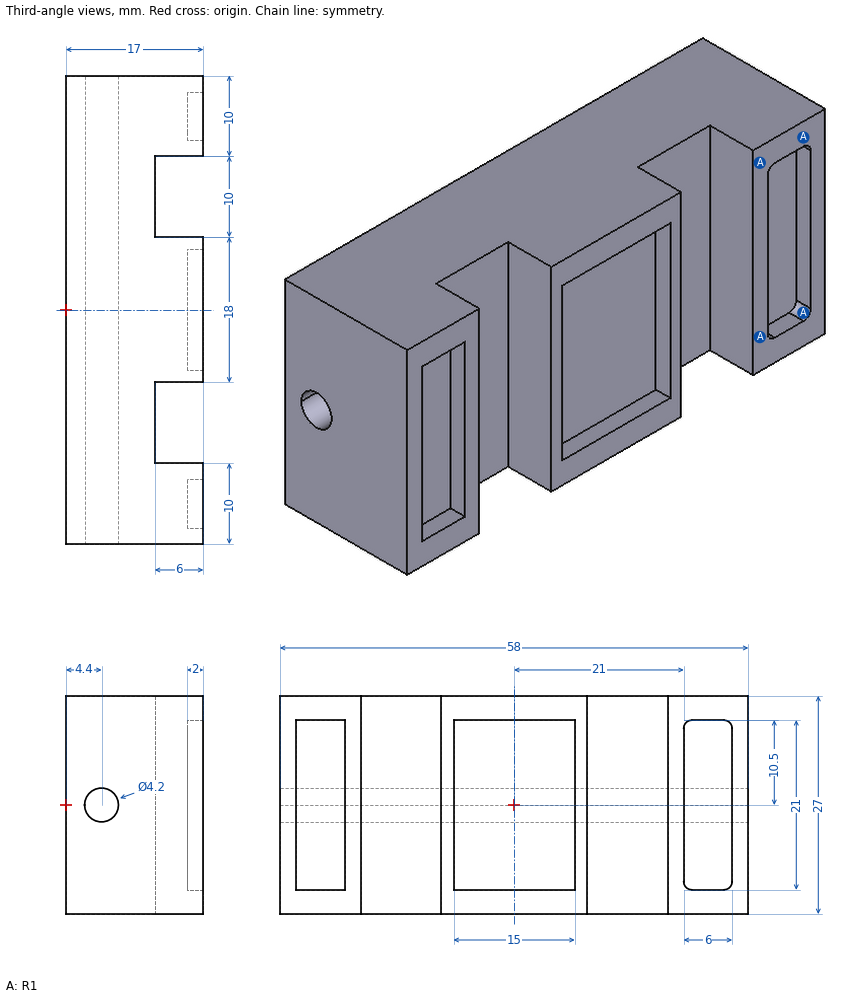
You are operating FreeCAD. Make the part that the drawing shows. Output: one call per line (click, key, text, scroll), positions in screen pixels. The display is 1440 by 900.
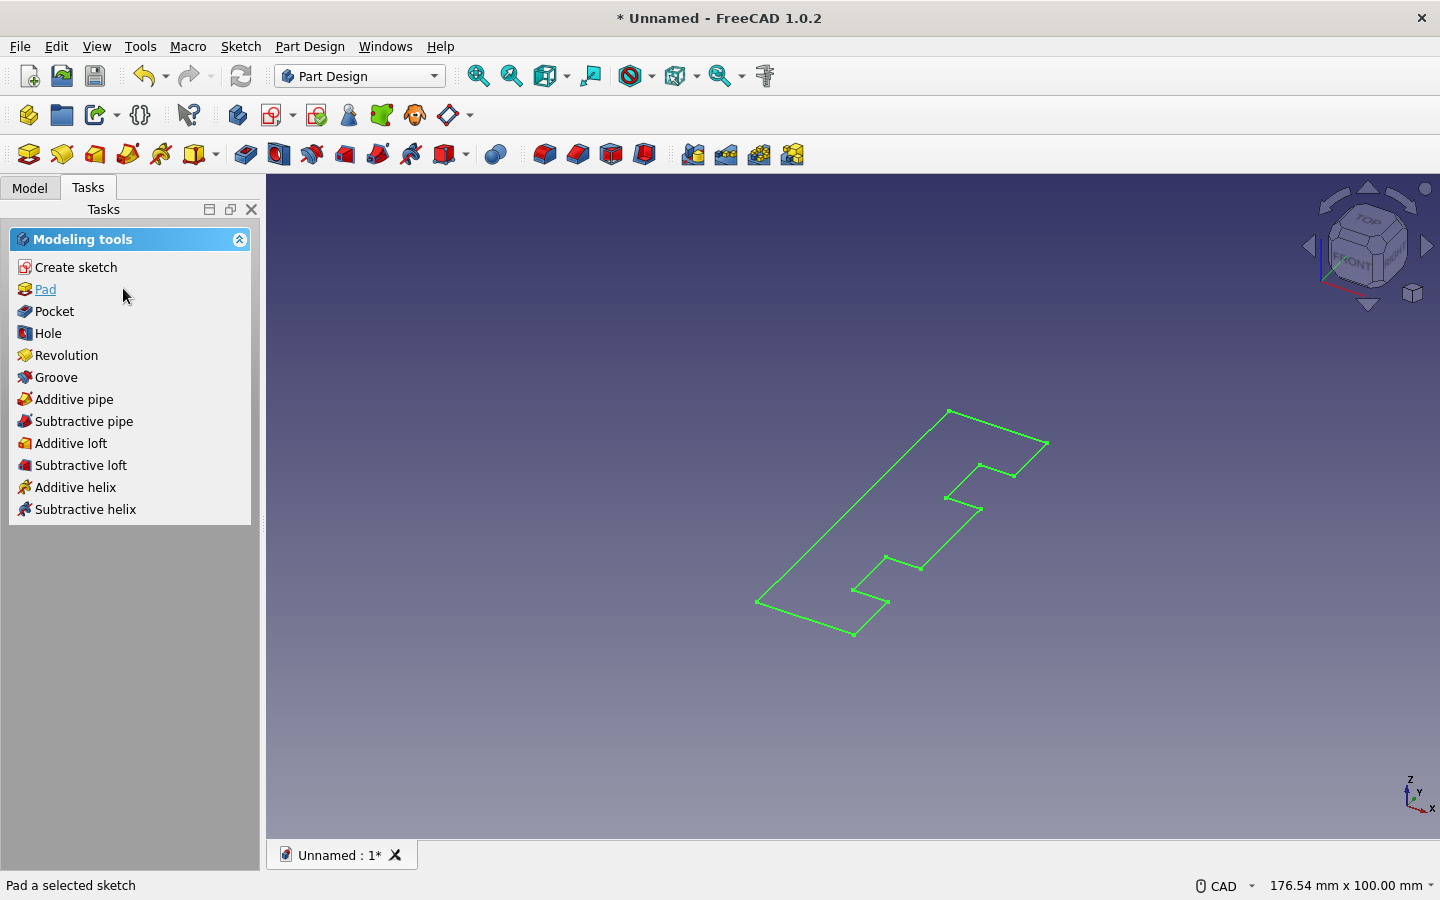
click(29, 154)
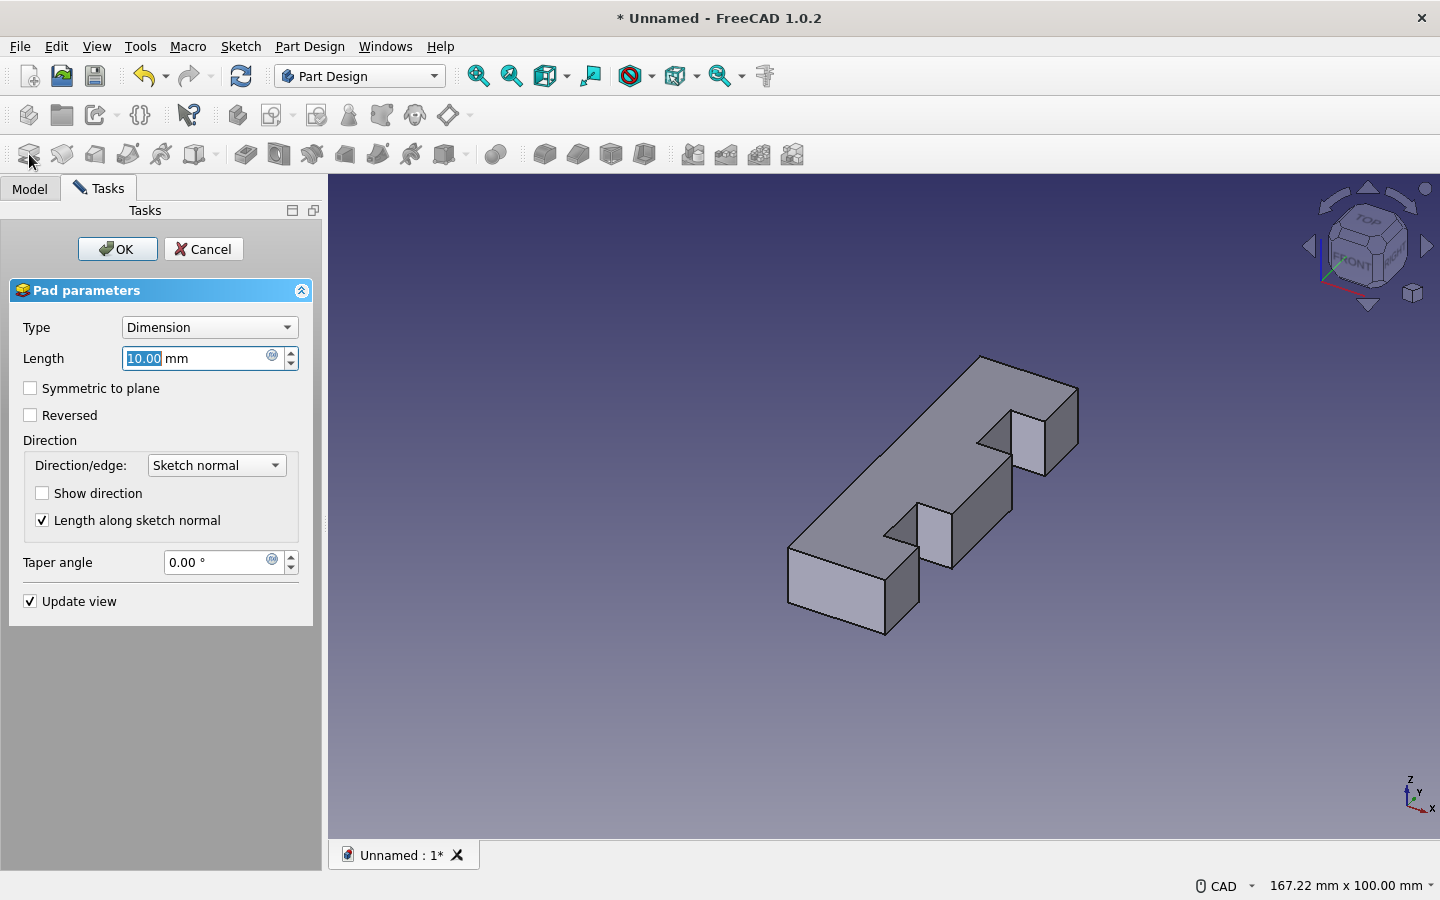
text(27)
key(Tab)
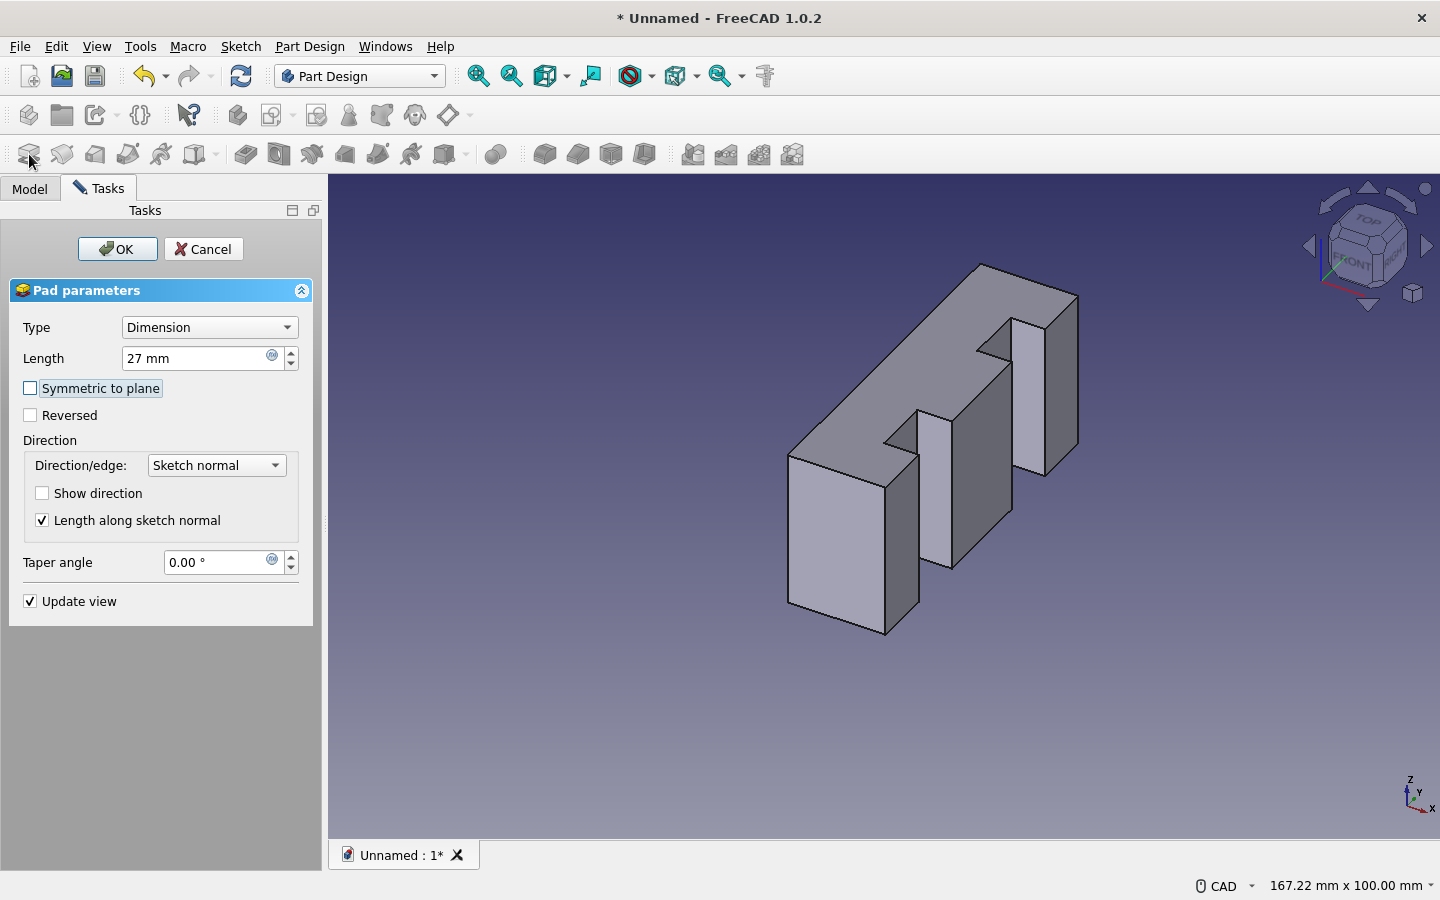
click(31, 388)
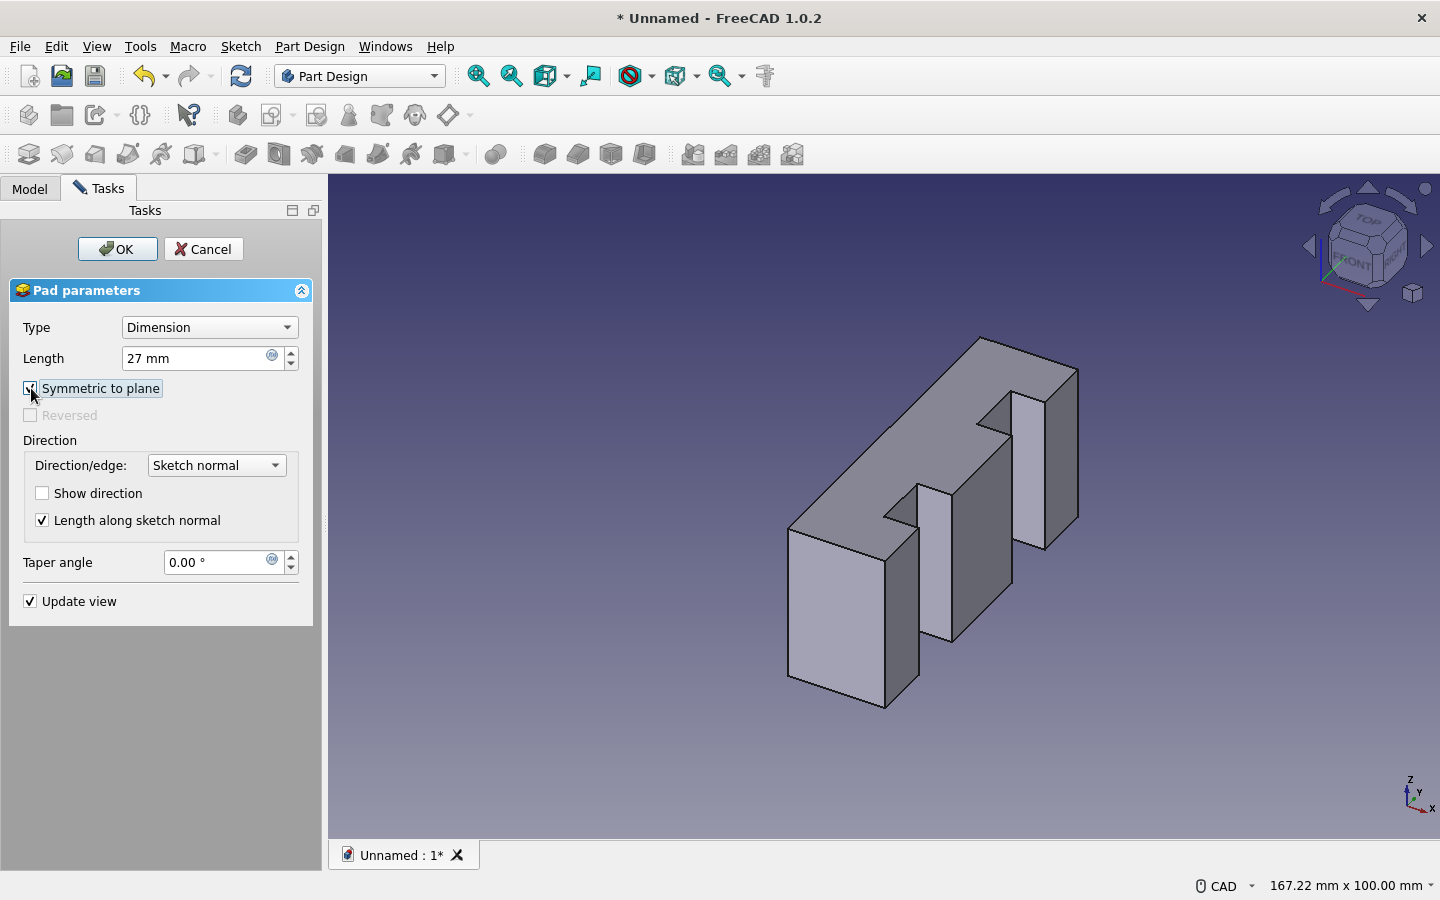
click(118, 249)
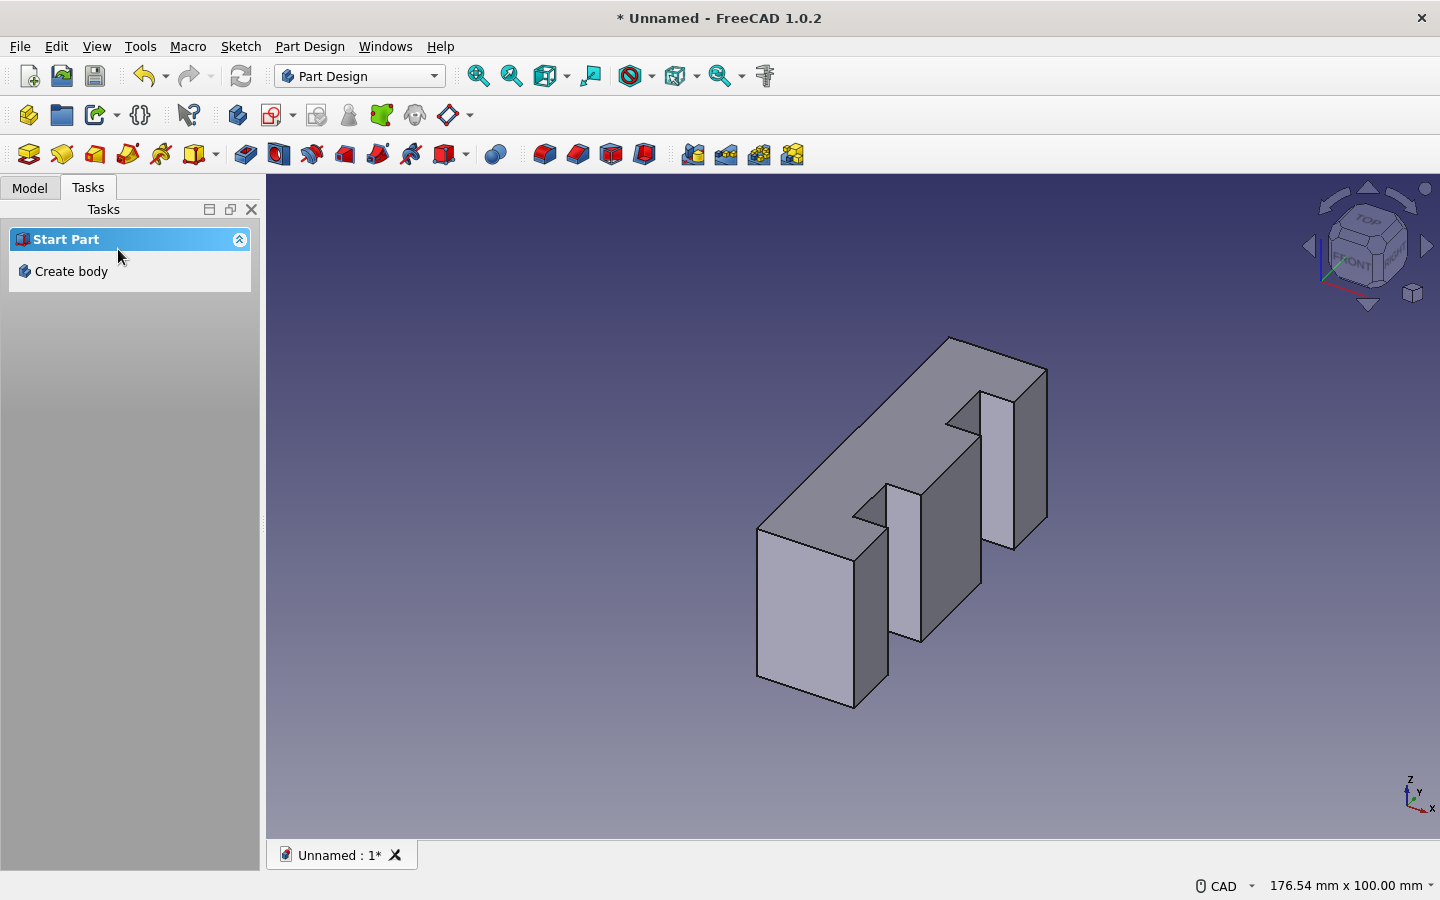
click(951, 517)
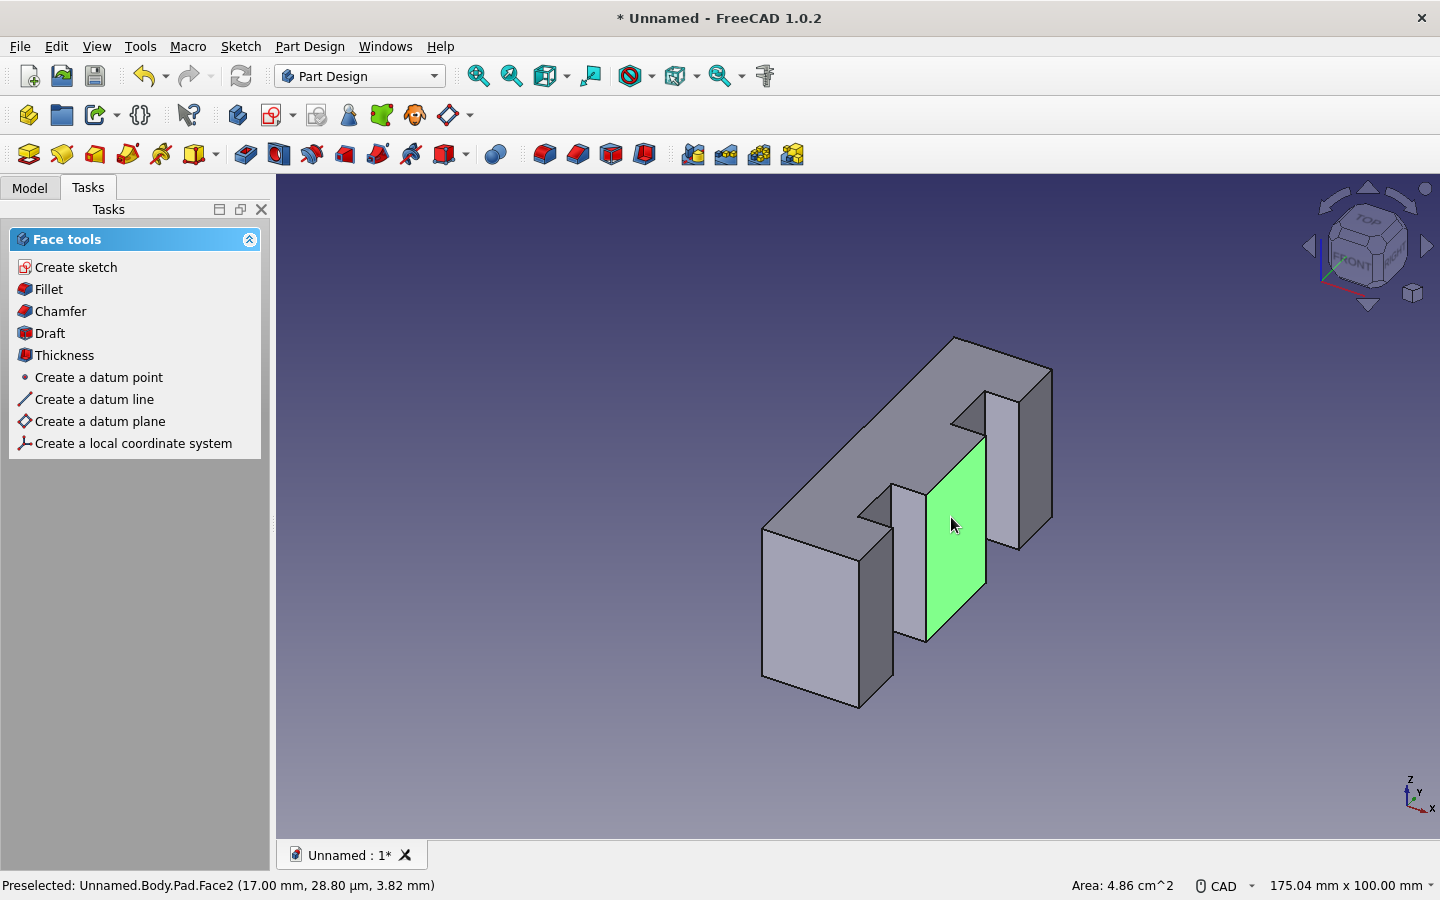
click(270, 116)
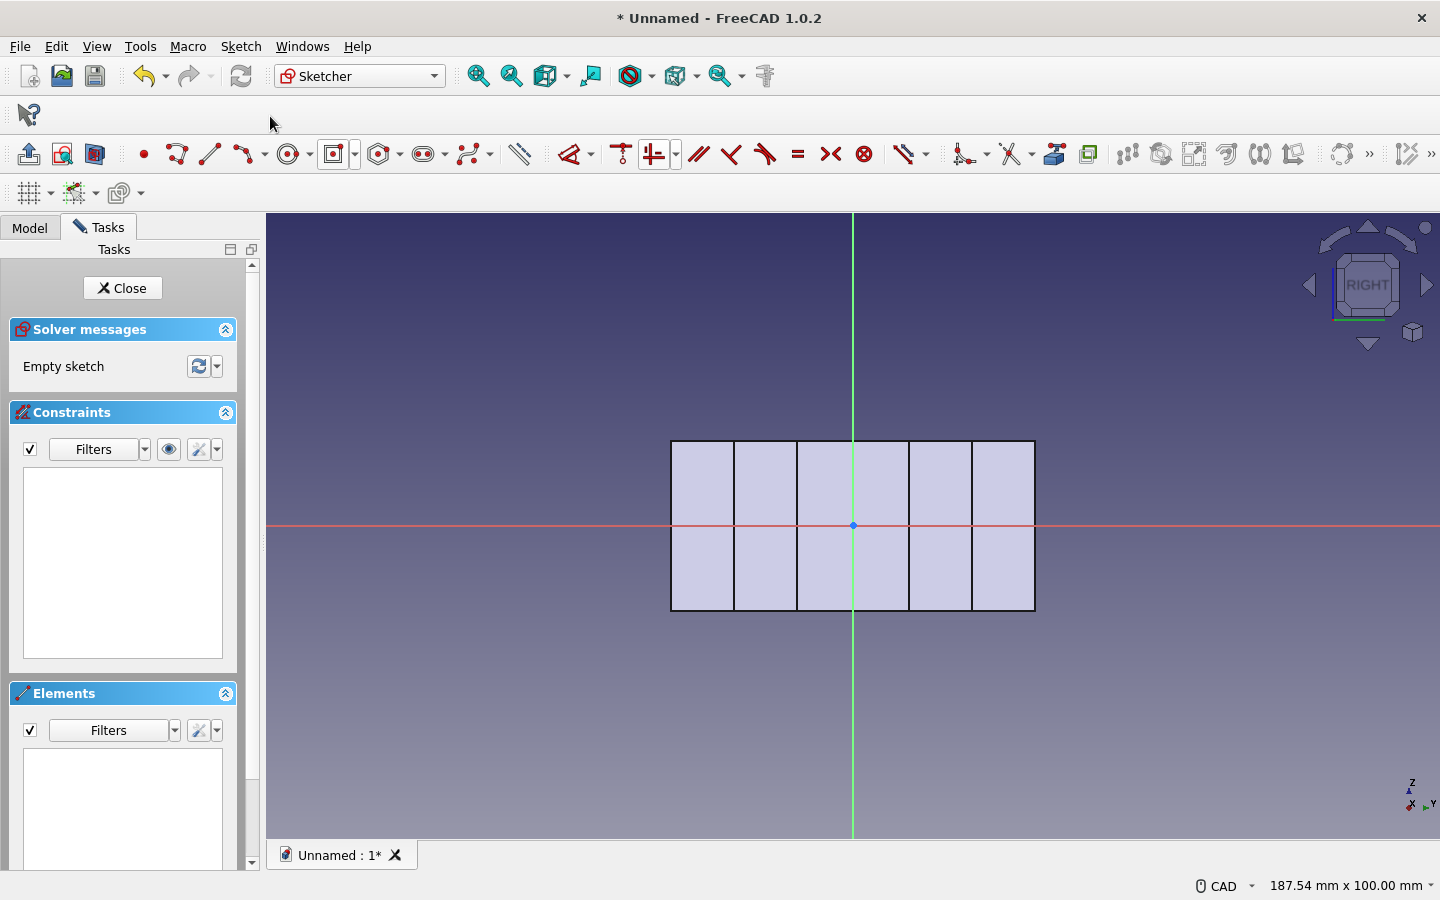
scroll(909, 526, up, 4)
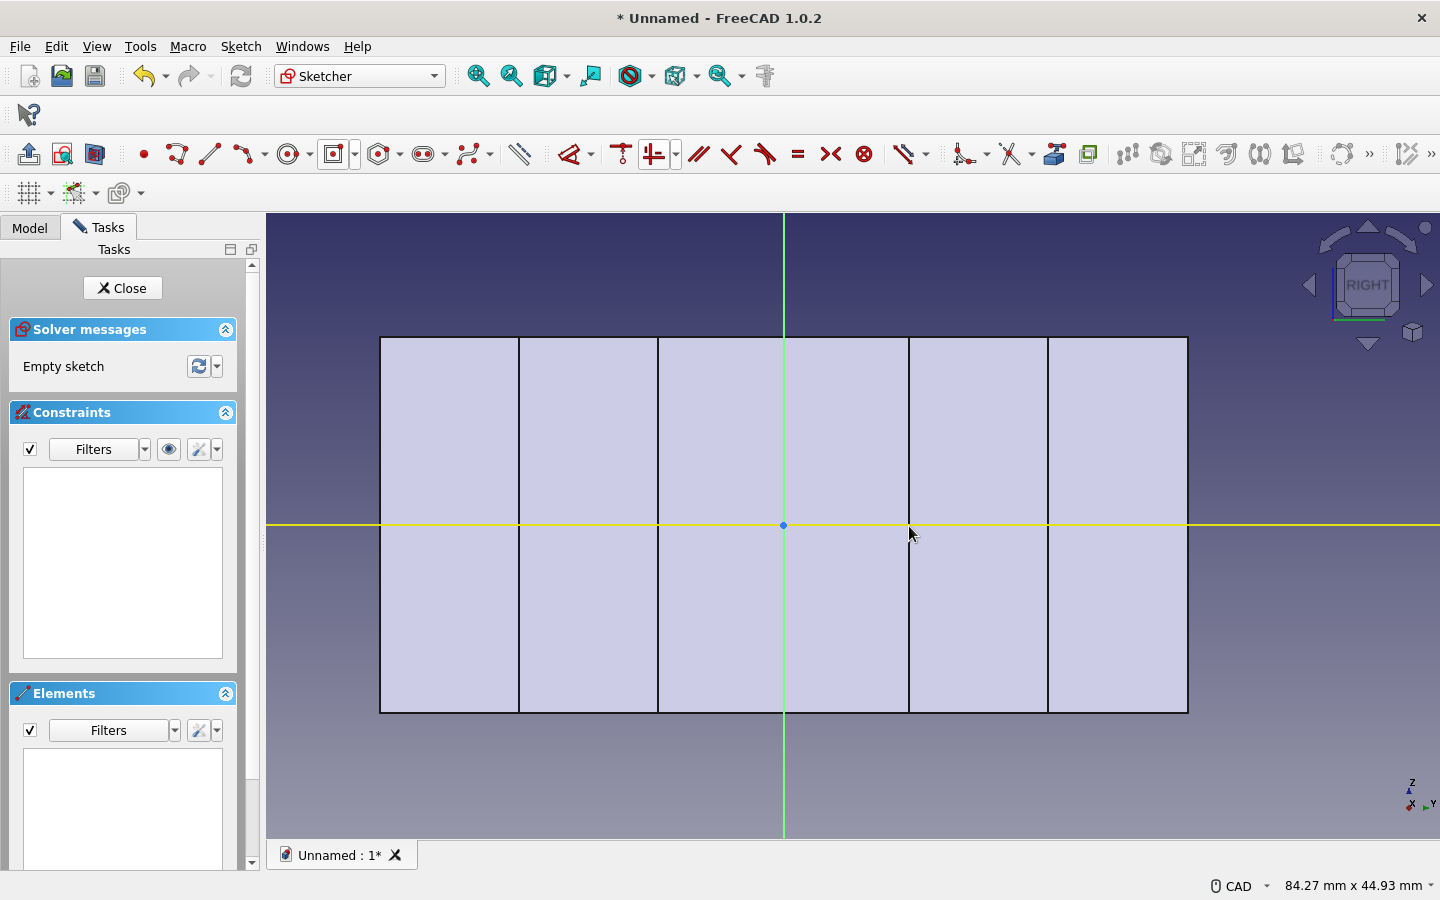
key(g)
key(r)